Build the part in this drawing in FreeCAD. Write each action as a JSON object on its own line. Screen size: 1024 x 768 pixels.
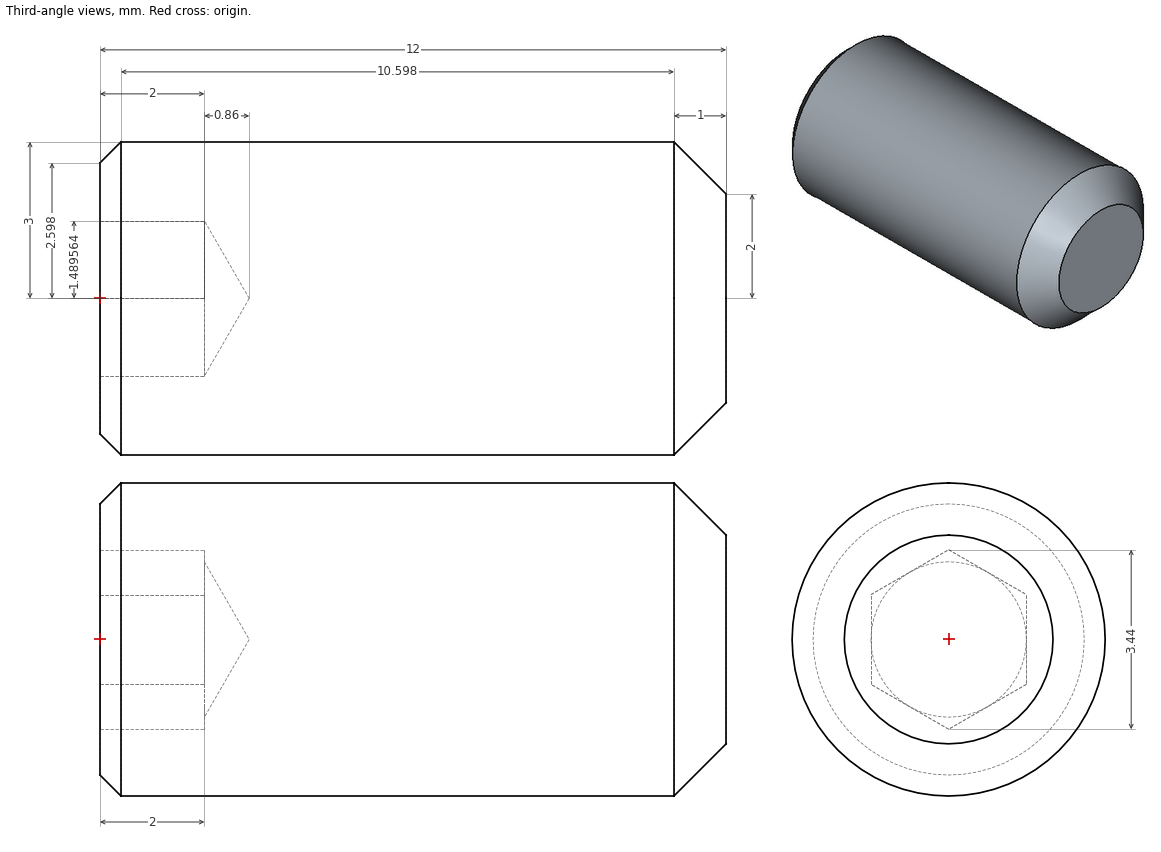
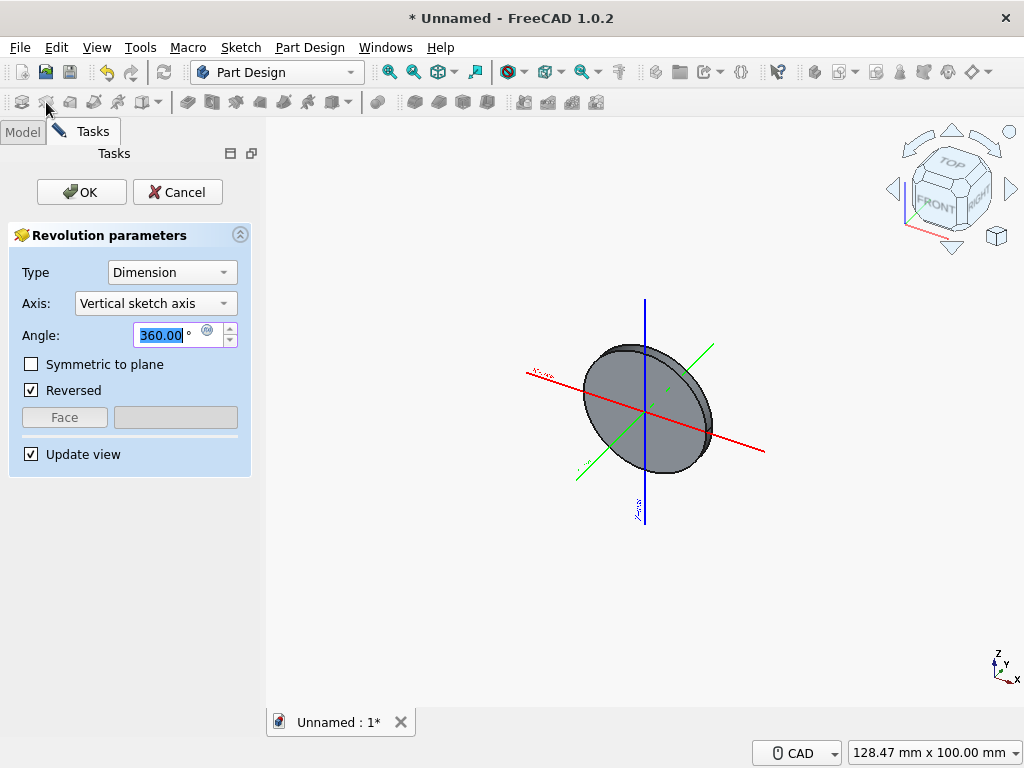
{"action": "left_click", "coordinate": [156, 304]}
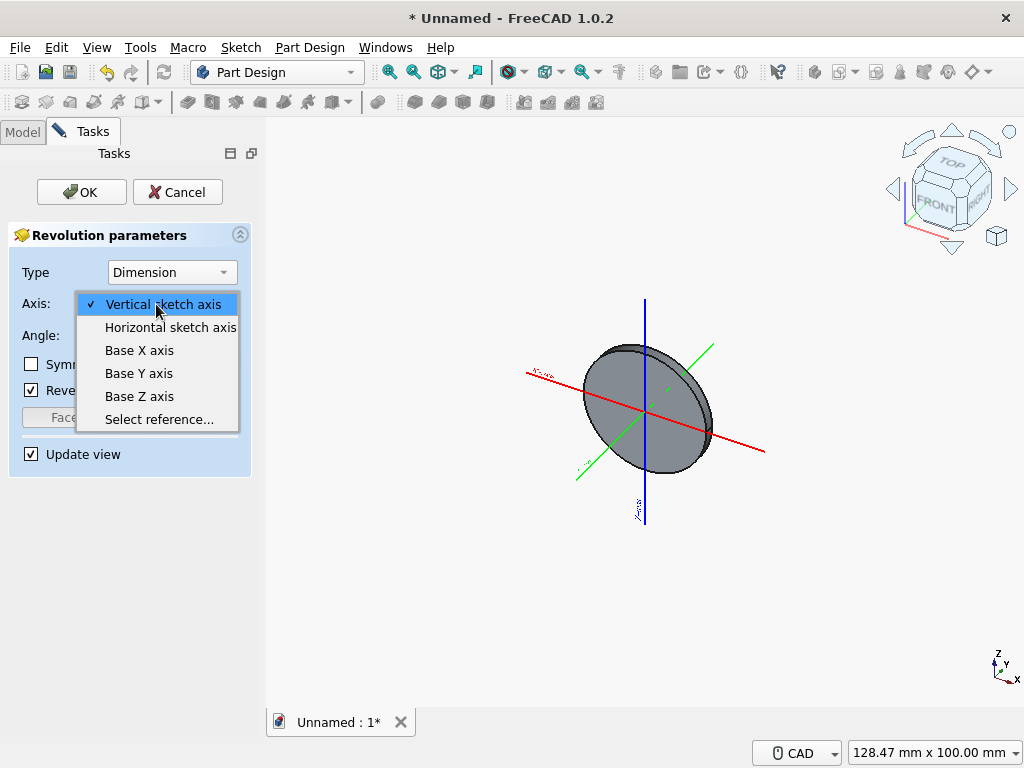
{"action": "left_click", "coordinate": [156, 328]}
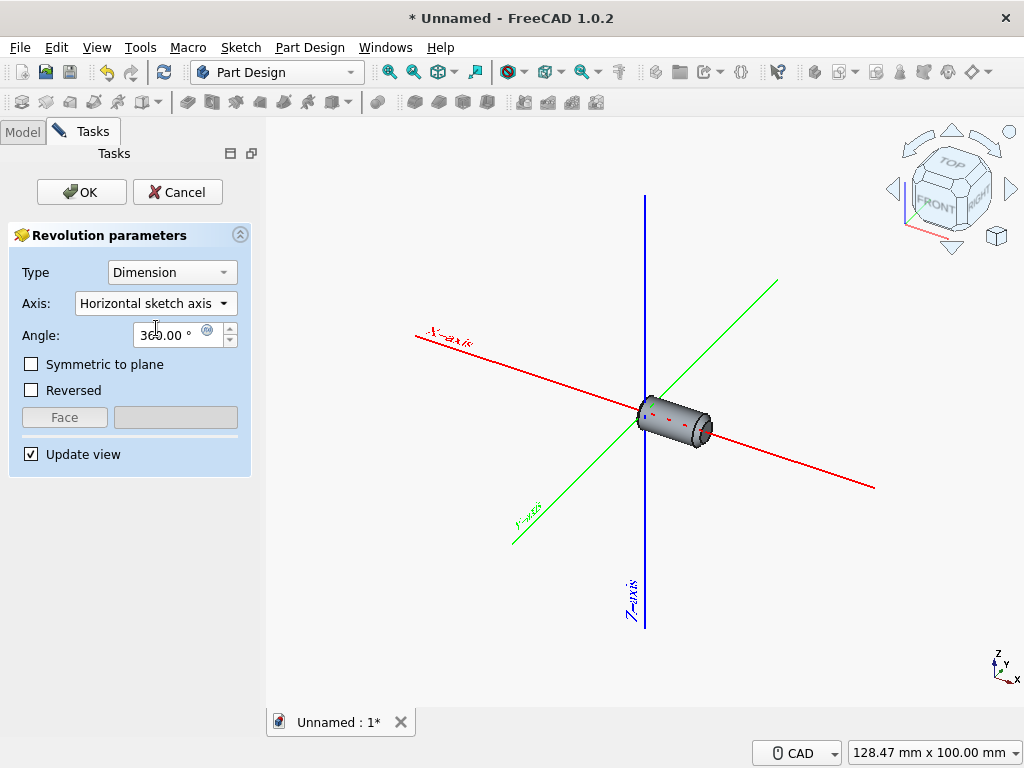
{"action": "left_click", "coordinate": [82, 192]}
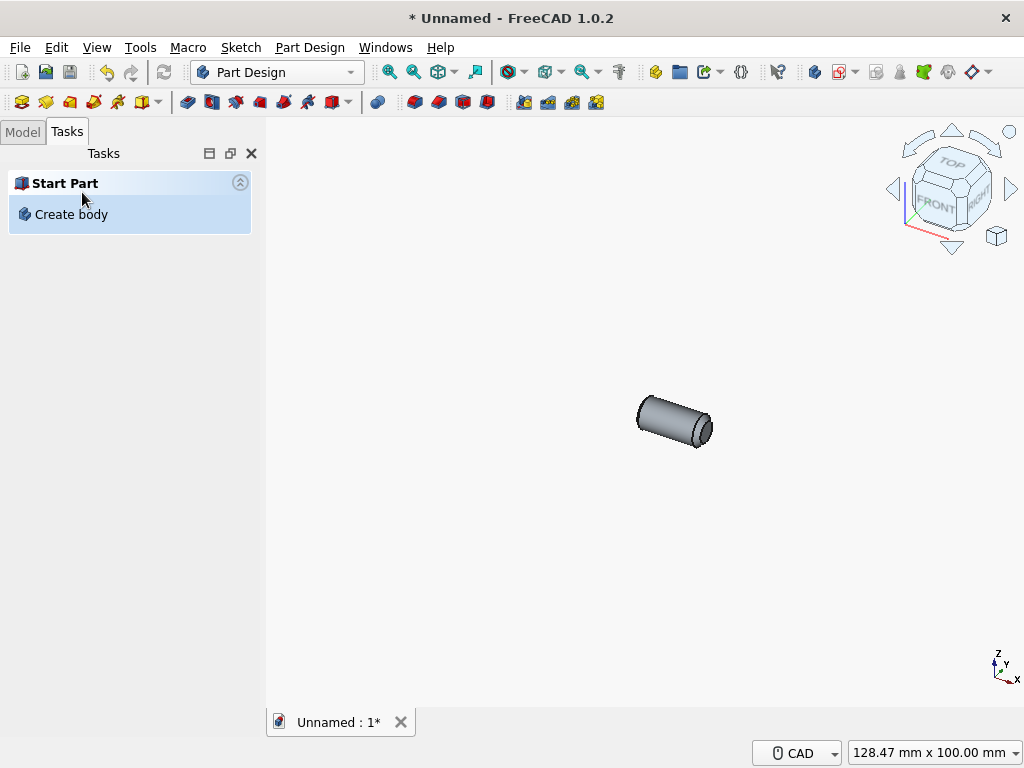
{"action": "left_click", "coordinate": [390, 72]}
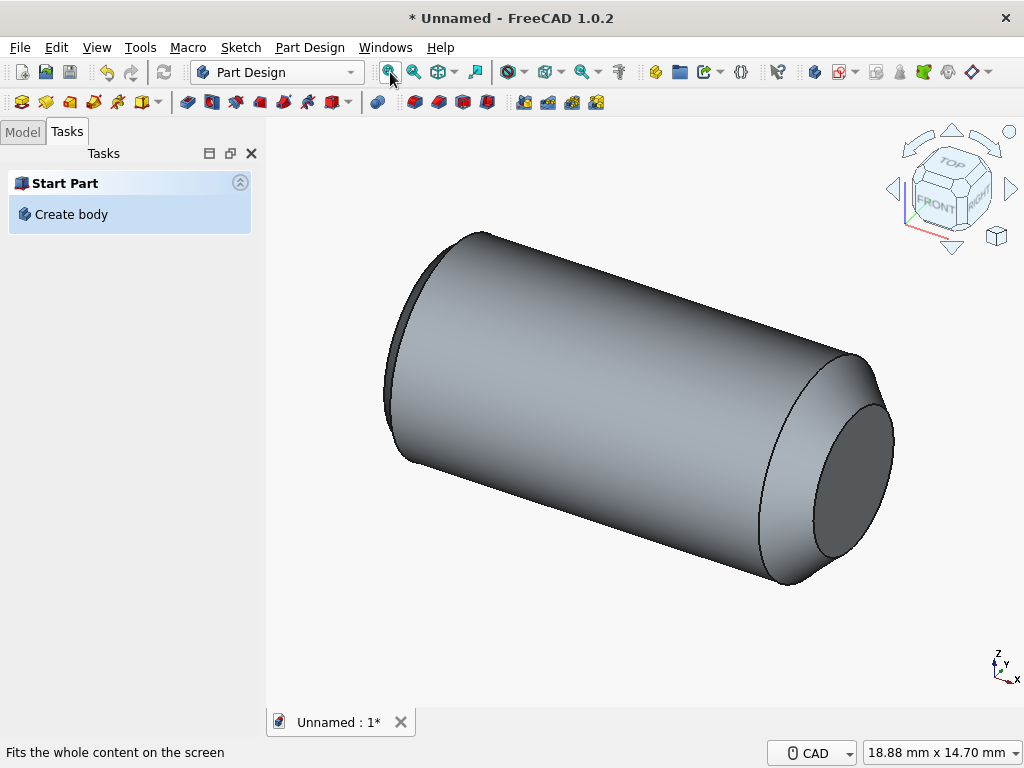
{"action": "key", "text": "6"}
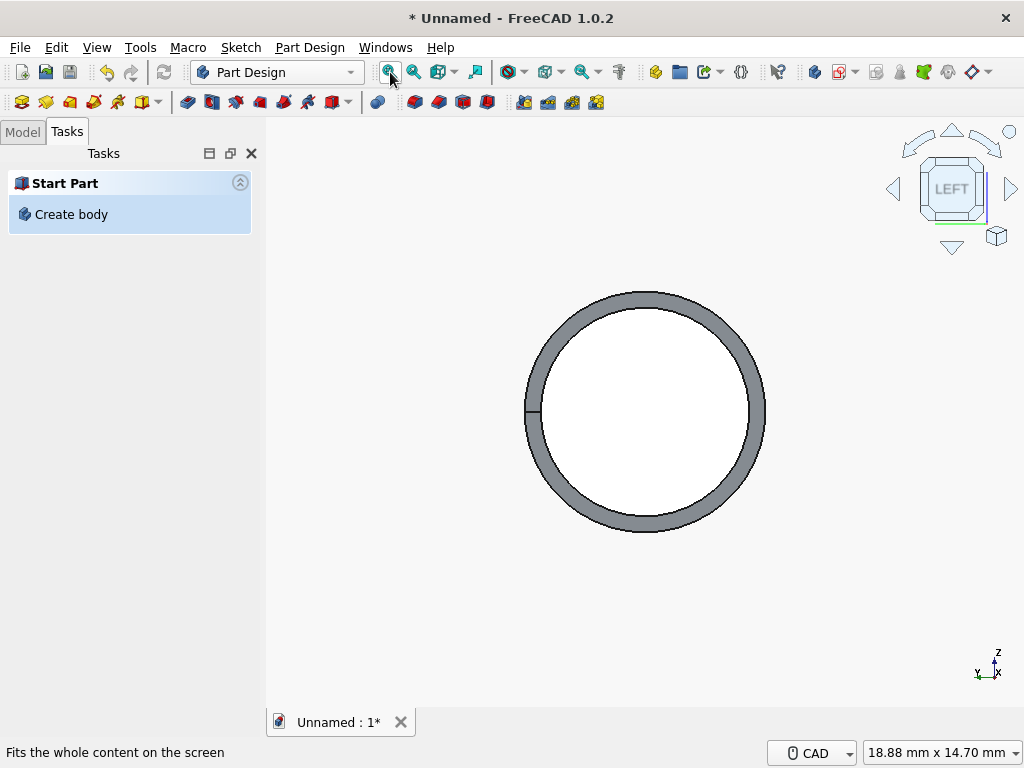
{"action": "left_click", "coordinate": [390, 72]}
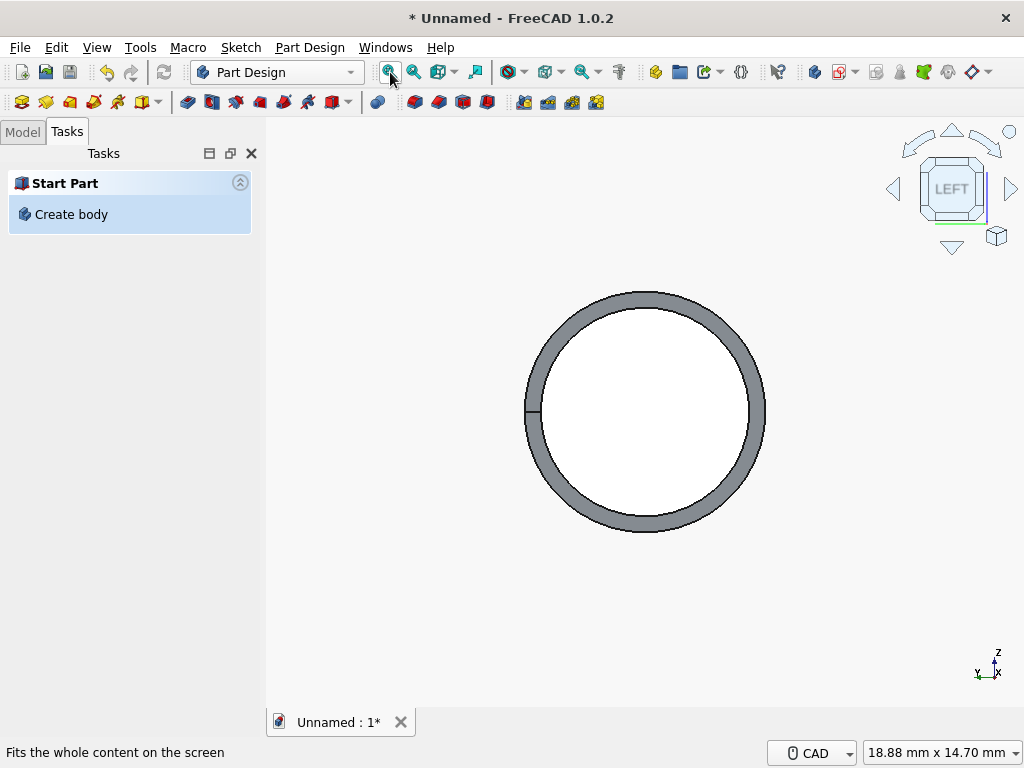
{"action": "left_click", "coordinate": [645, 411]}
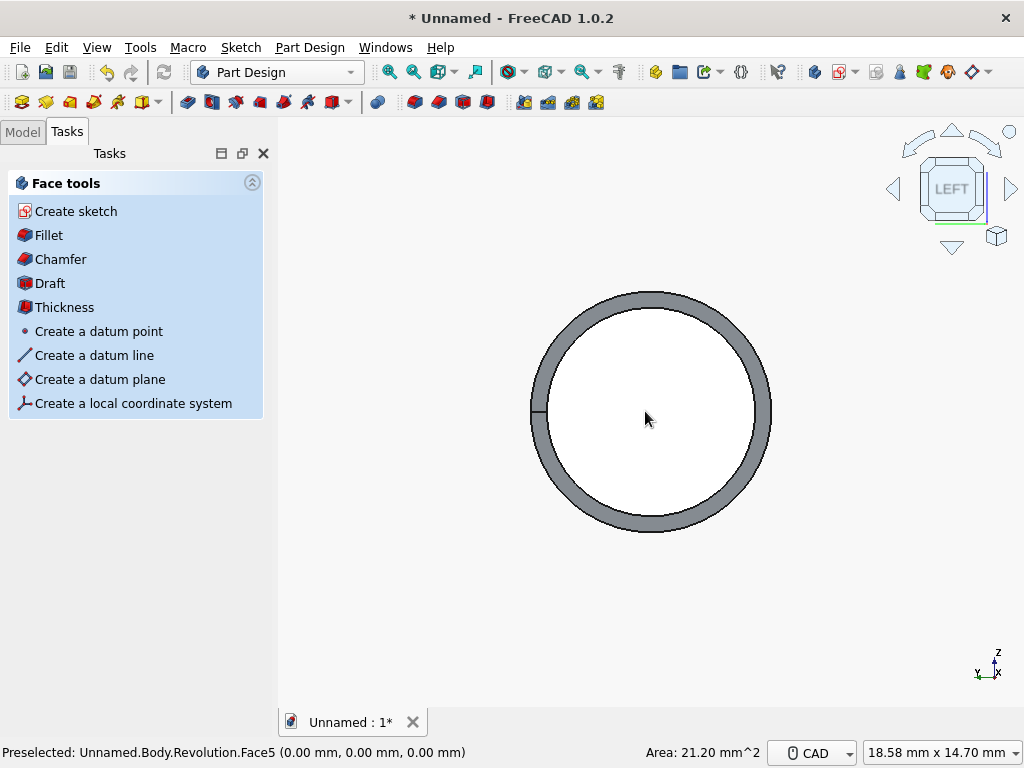
{"action": "left_click", "coordinate": [840, 72]}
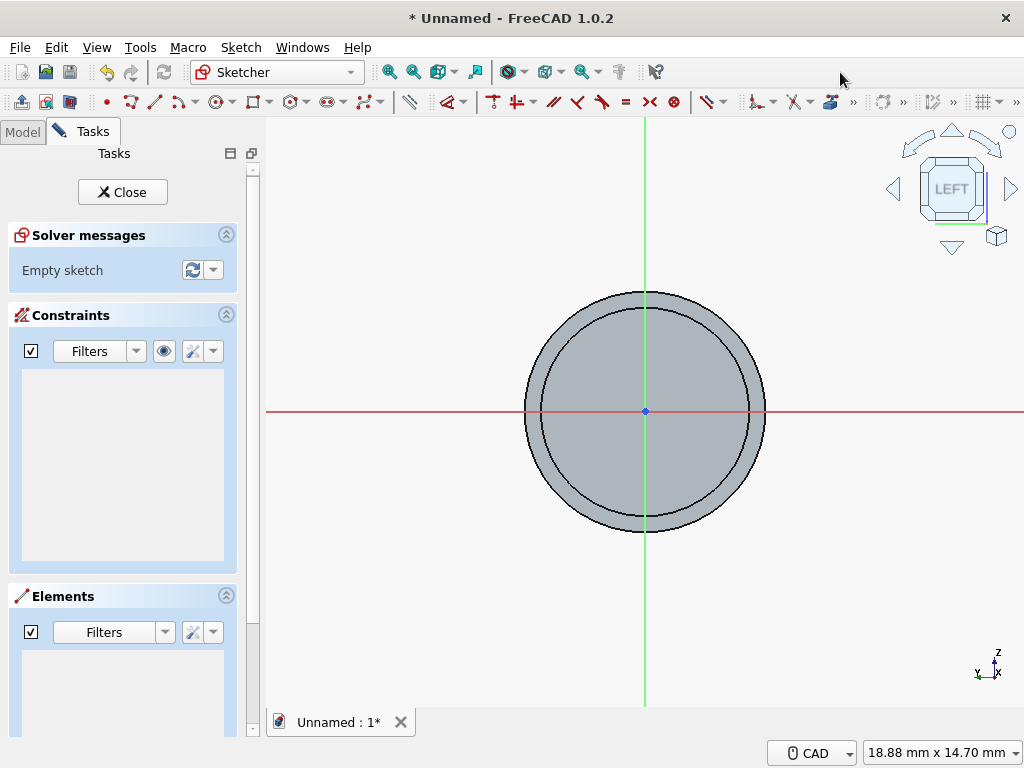
{"action": "scroll", "coordinate": [685, 412], "scroll_direction": "up", "scroll_amount": 5}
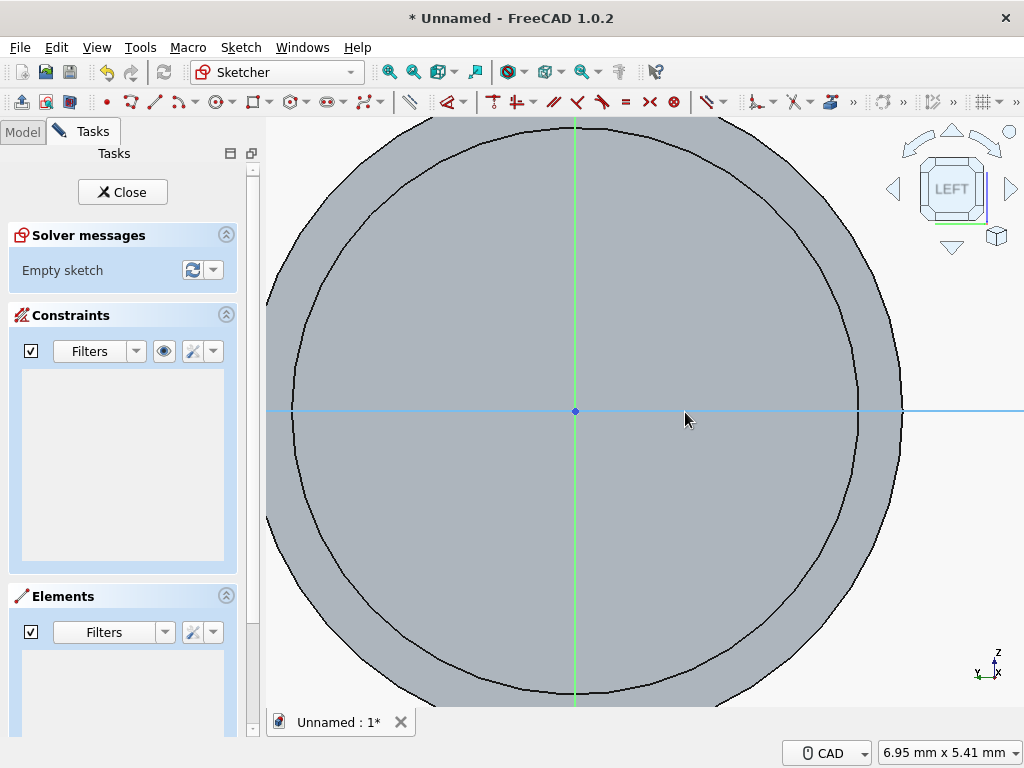
{"action": "key", "text": "g p 6"}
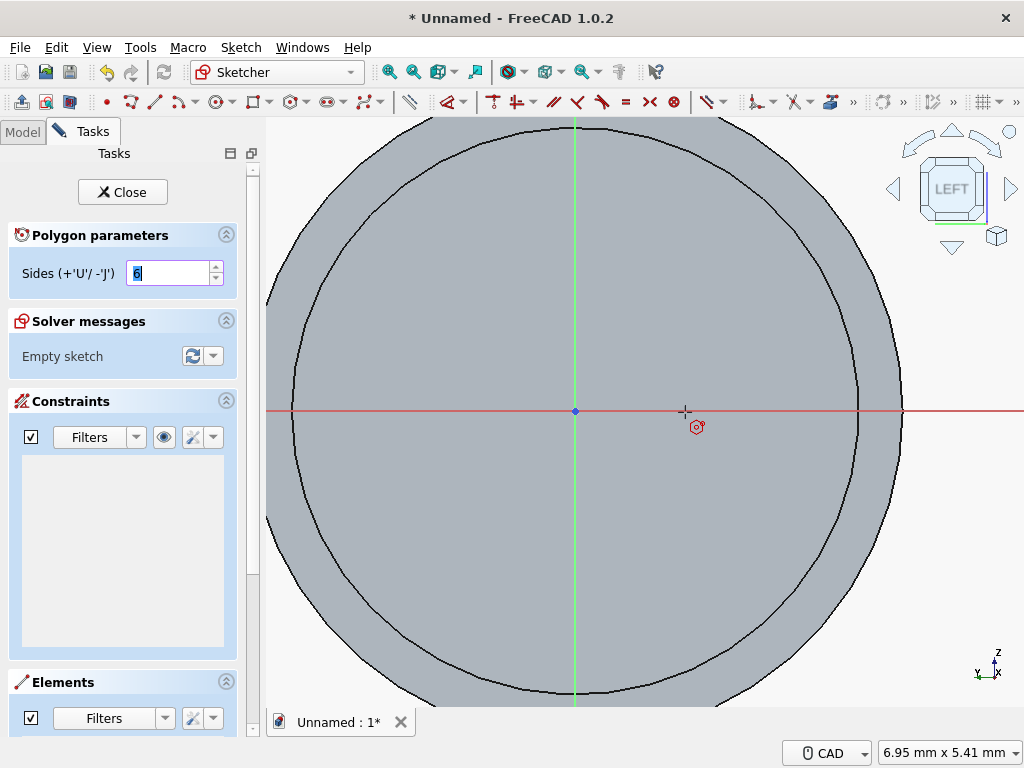
{"action": "left_click", "coordinate": [575, 411]}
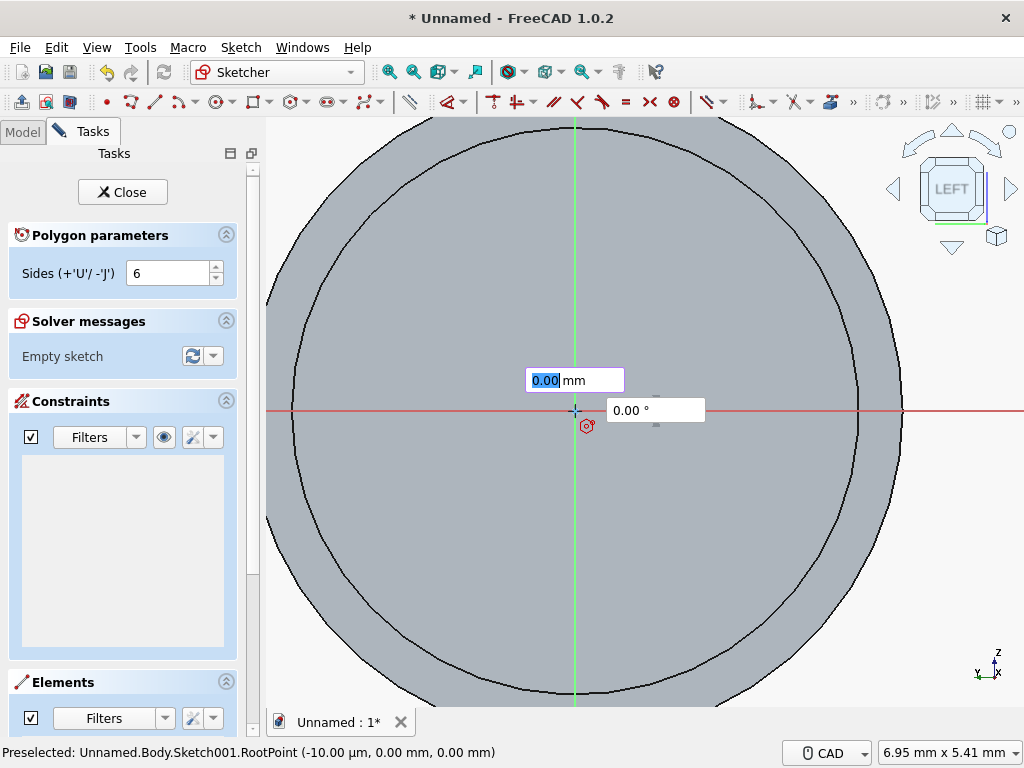
{"action": "left_click", "coordinate": [575, 223]}
{"action": "right_click", "coordinate": [575, 223]}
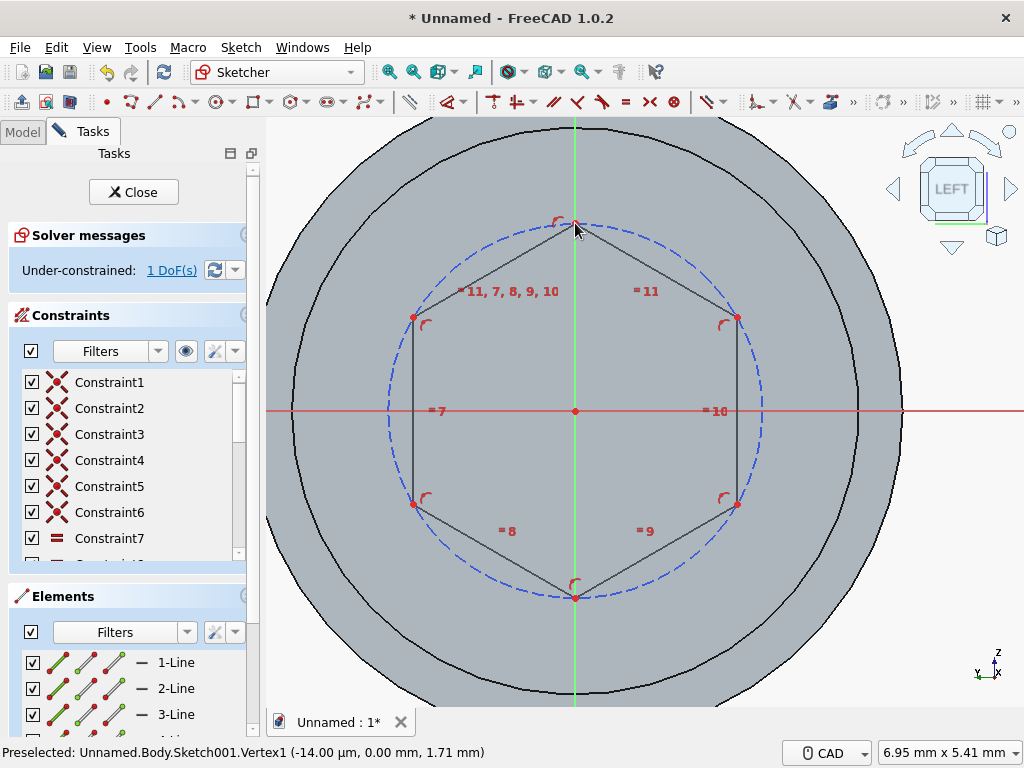
{"action": "key", "text": "d"}